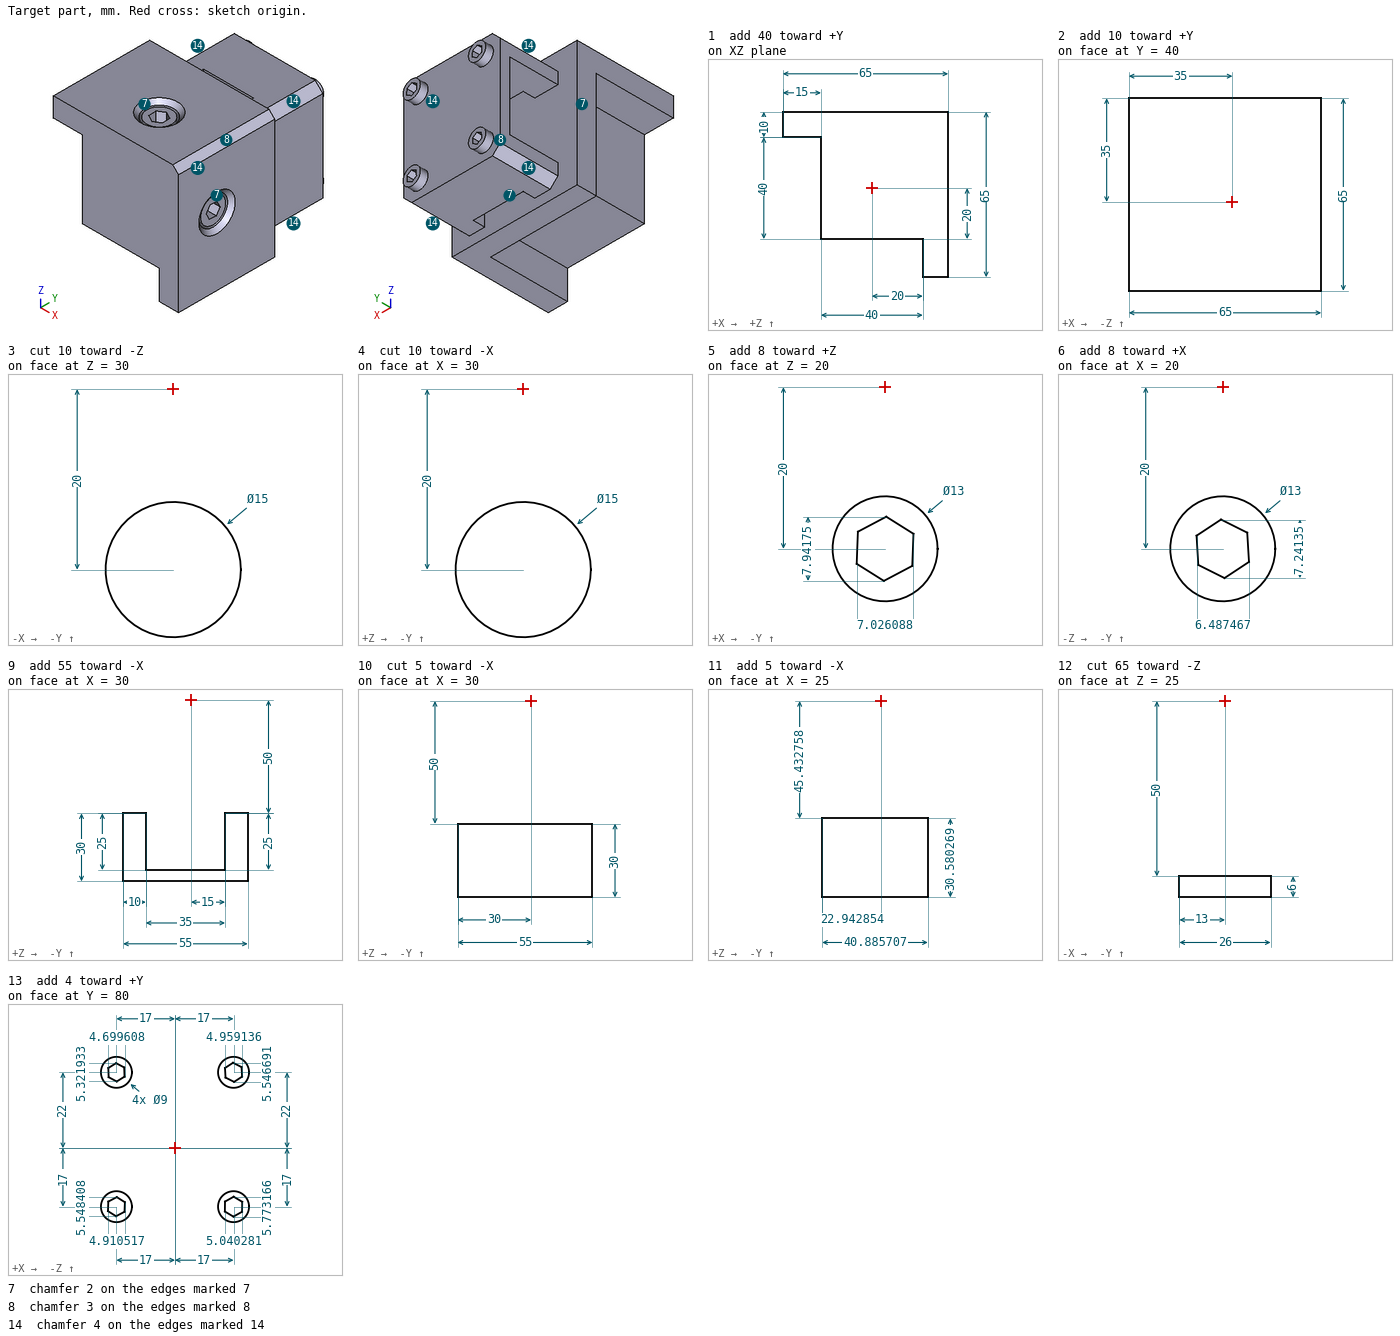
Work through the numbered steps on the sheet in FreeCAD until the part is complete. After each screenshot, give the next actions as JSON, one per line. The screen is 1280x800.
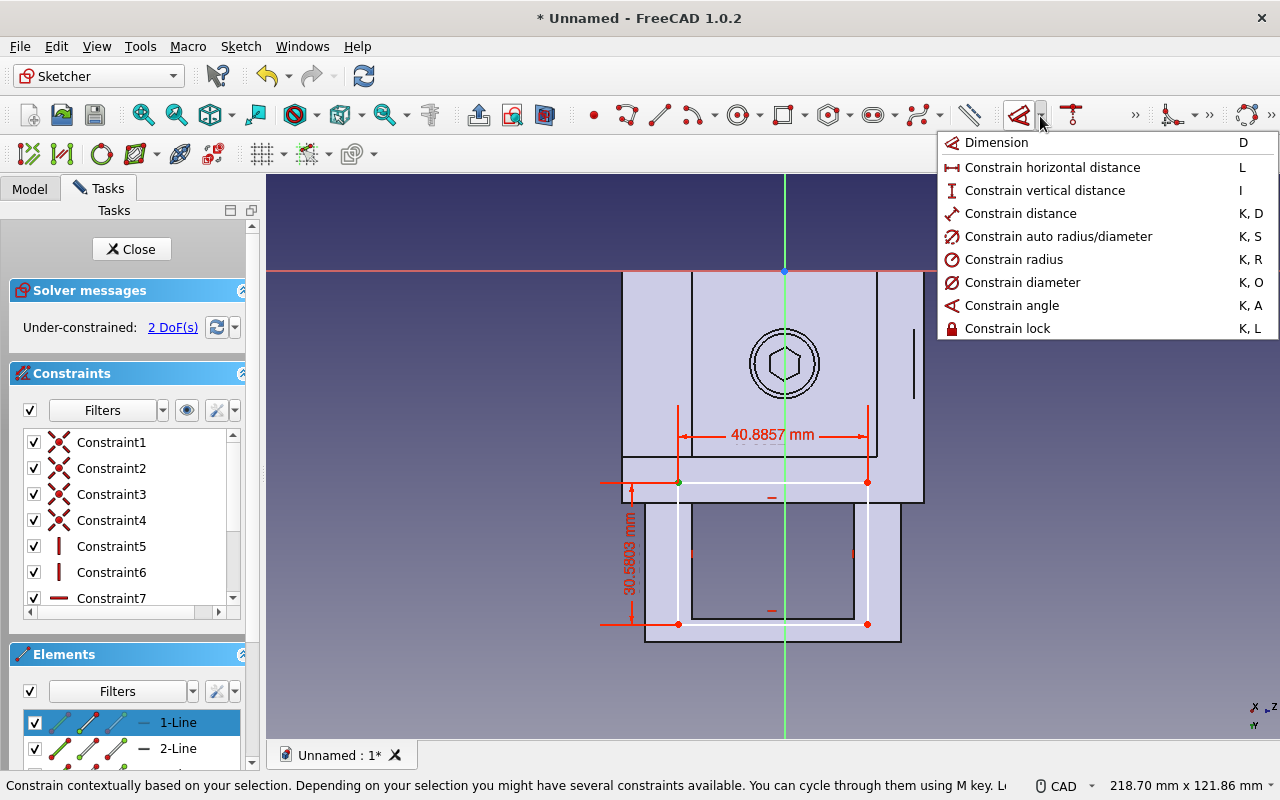
{"action": "left_click", "coordinate": [1108, 168]}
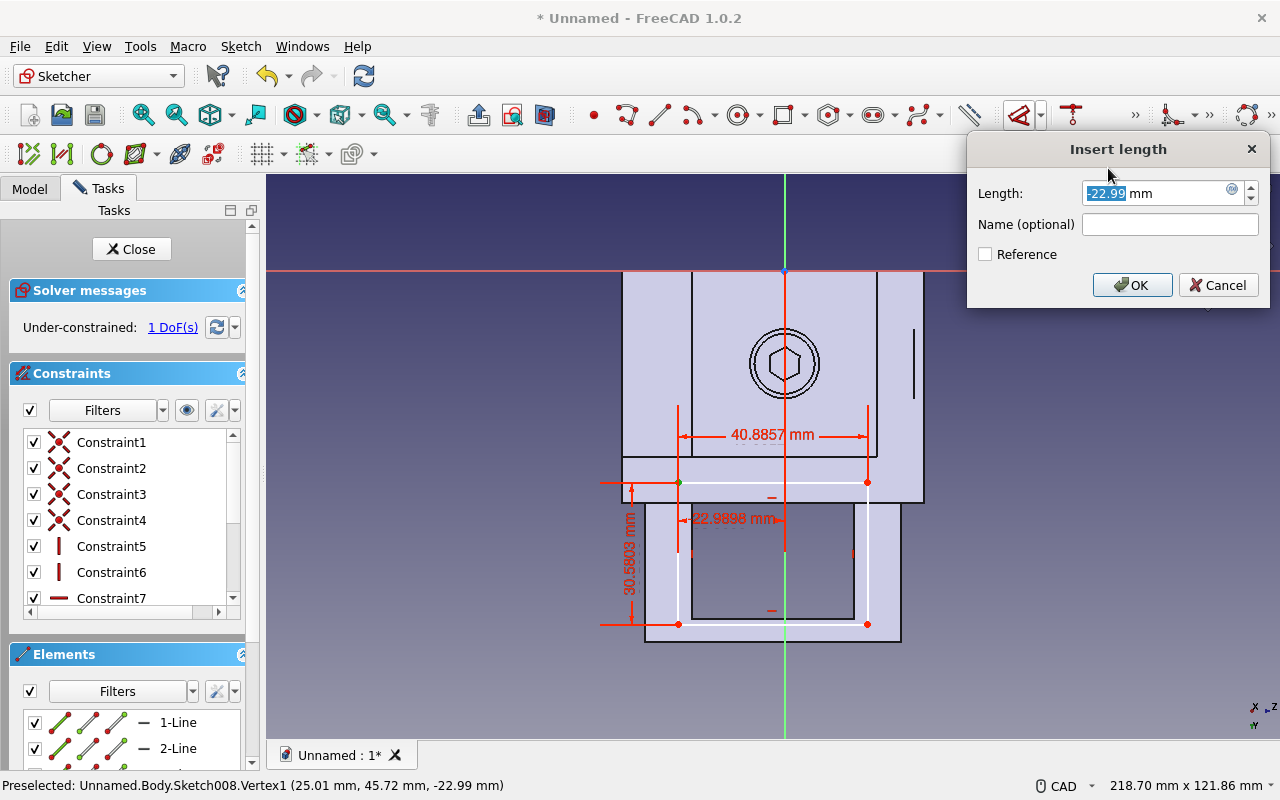
{"action": "type", "text": "-22.942854"}
{"action": "key", "text": "Return"}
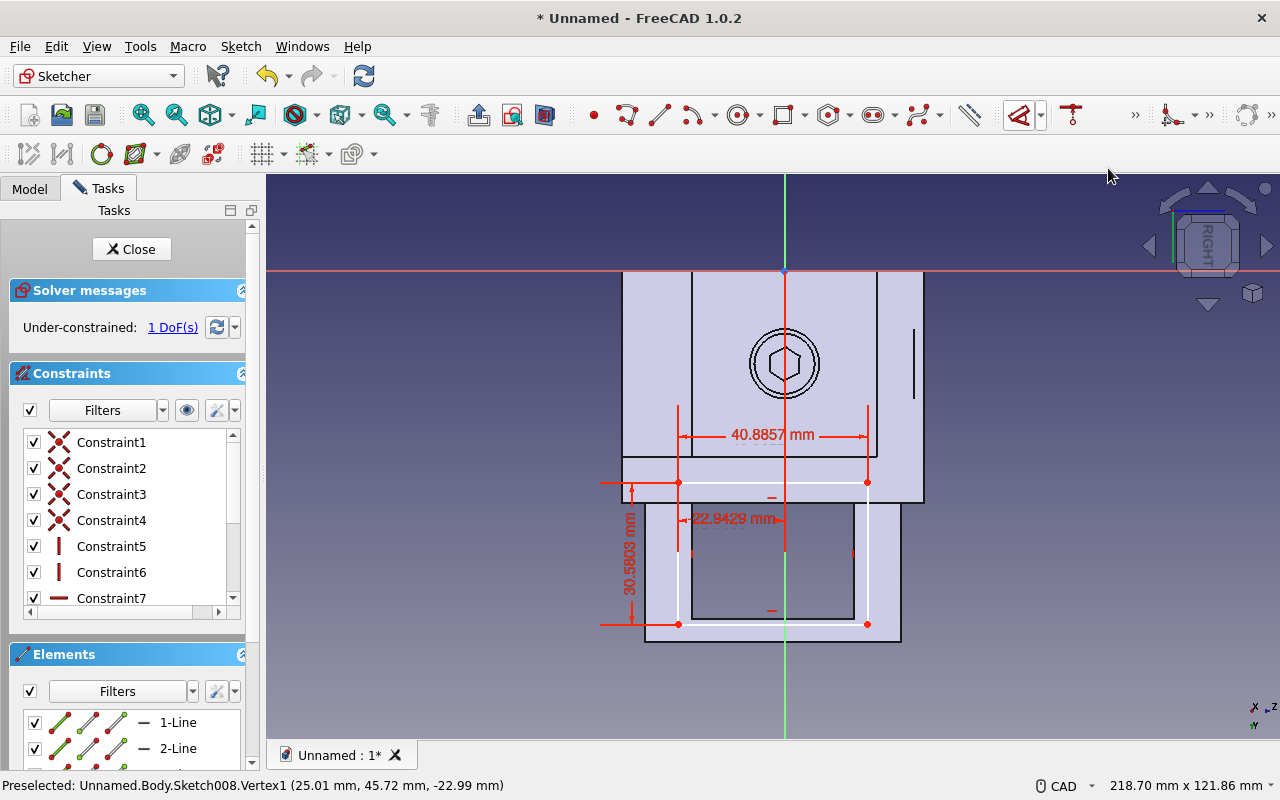
{"action": "left_click", "coordinate": [678, 483]}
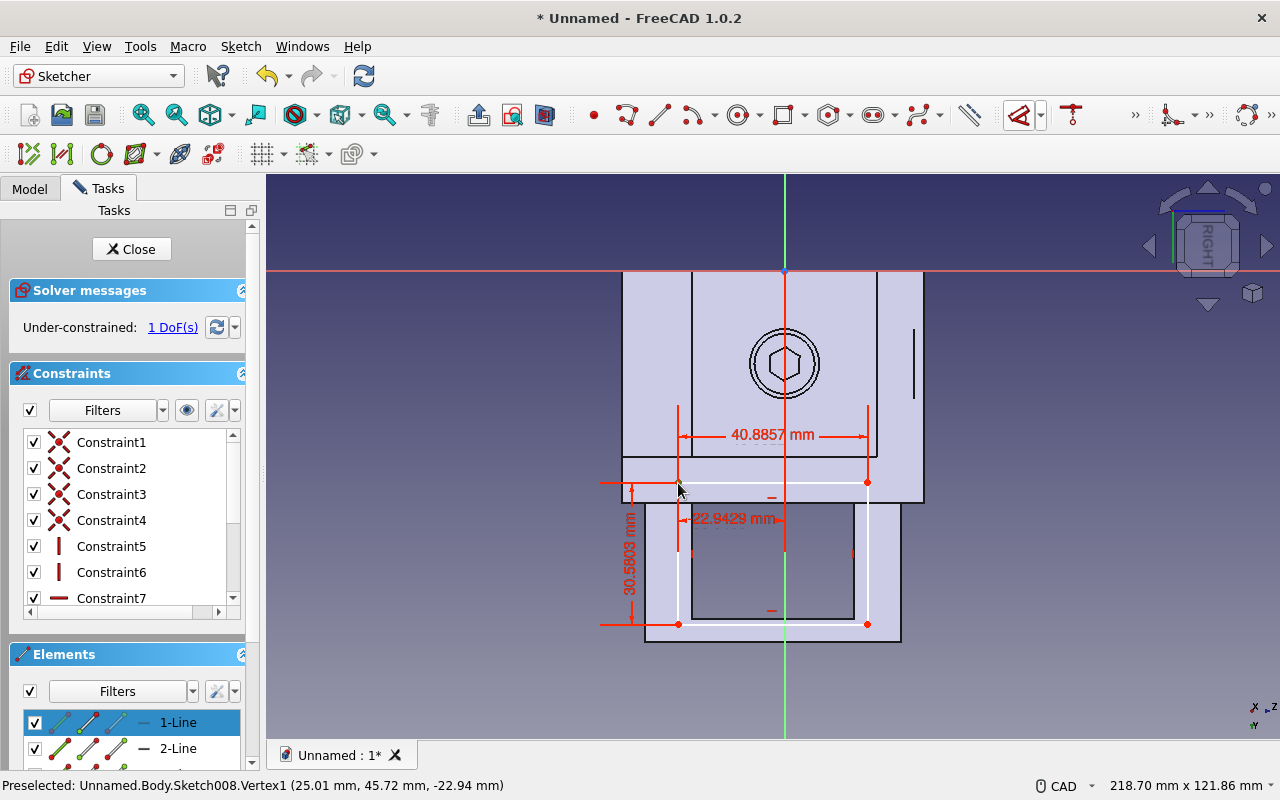
{"action": "left_click", "coordinate": [1040, 116]}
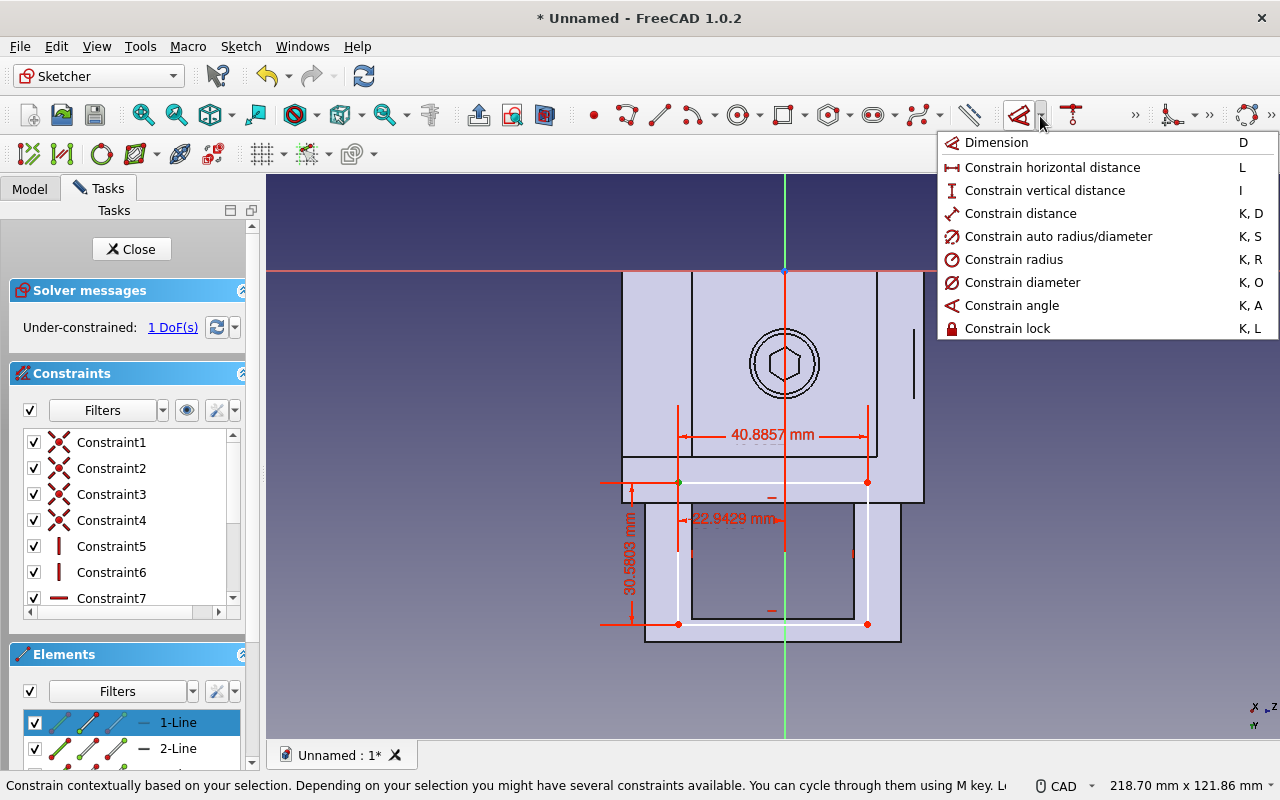
{"action": "left_click", "coordinate": [1108, 190]}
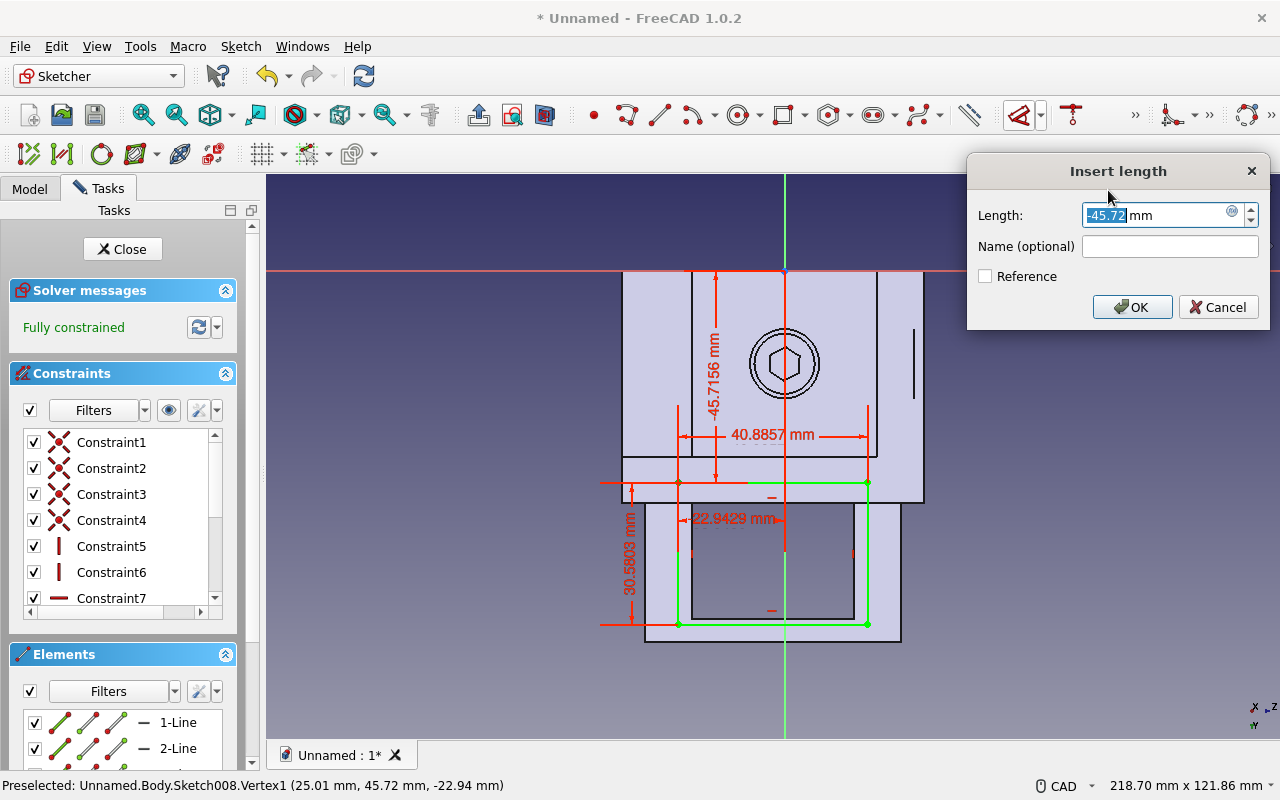
{"action": "type", "text": "-45.432758"}
{"action": "key", "text": "Return"}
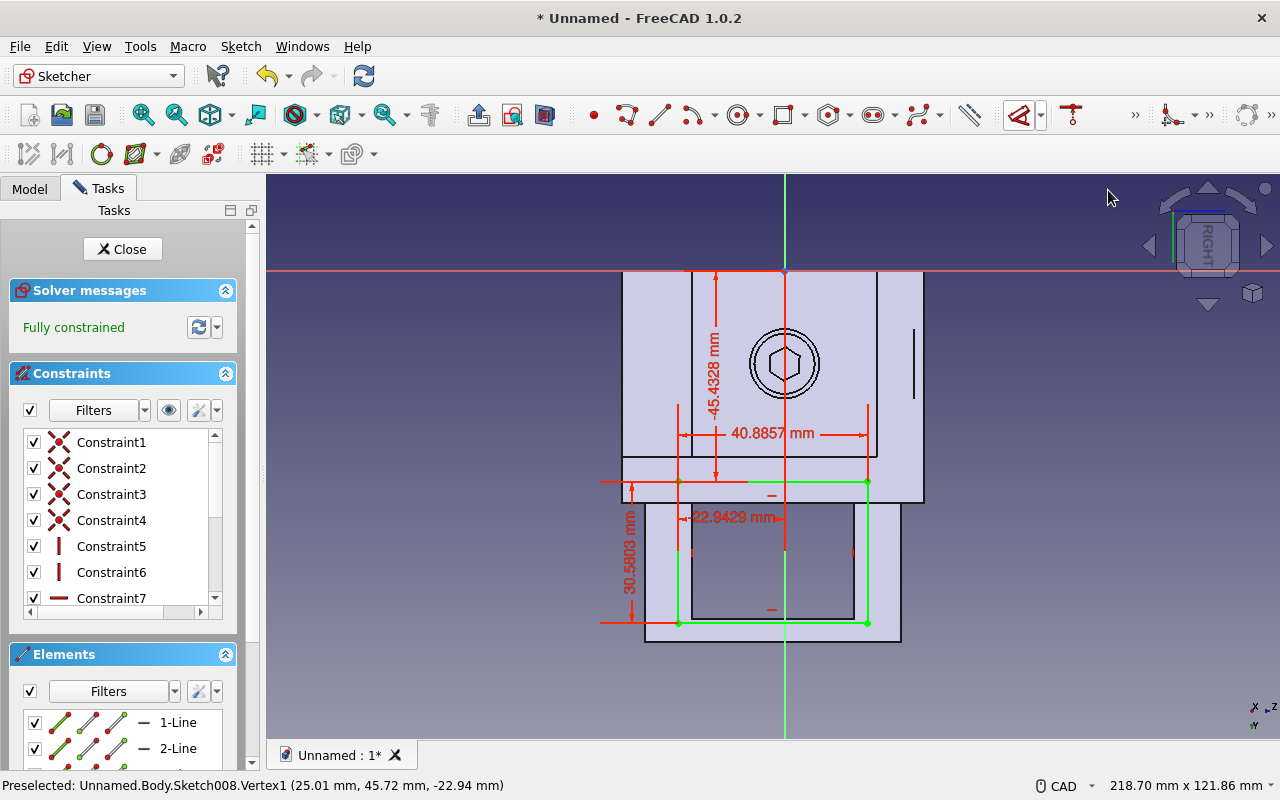
{"action": "left_click", "coordinate": [123, 249]}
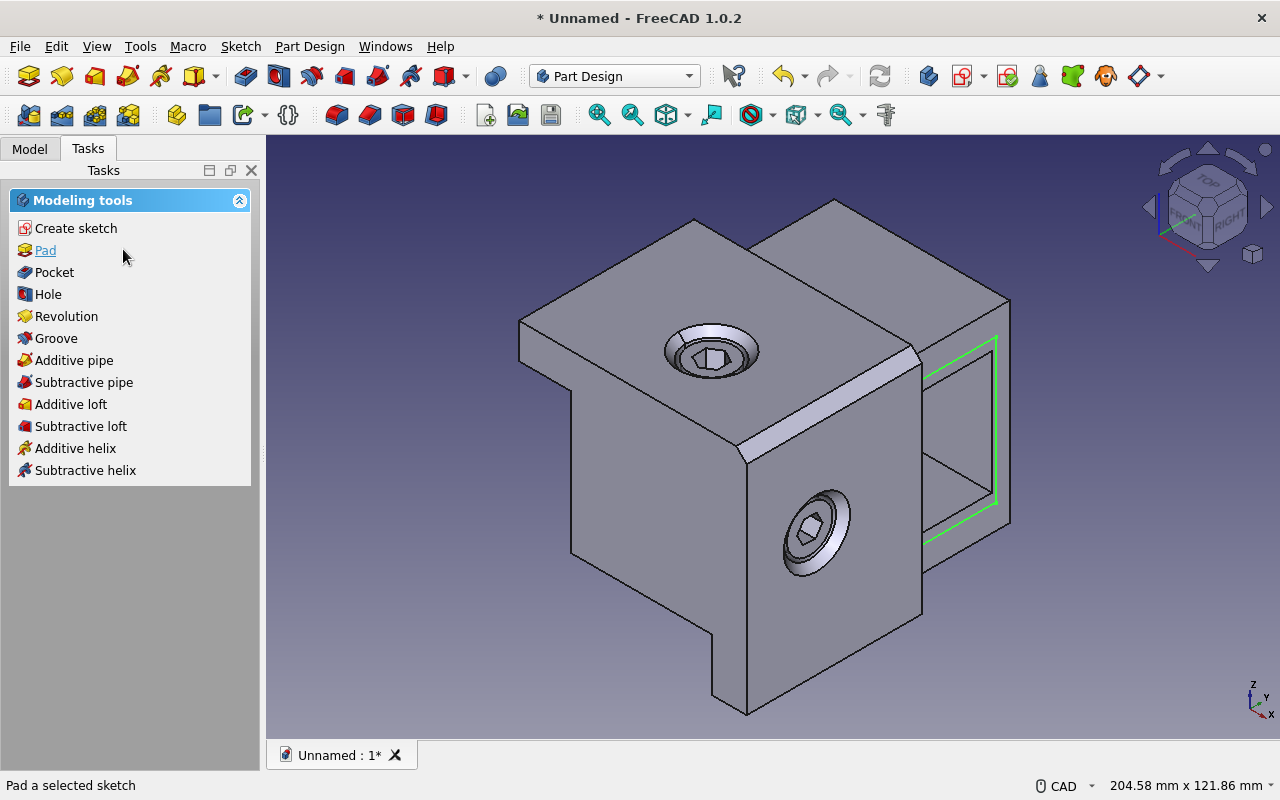
{"action": "left_click", "coordinate": [29, 76]}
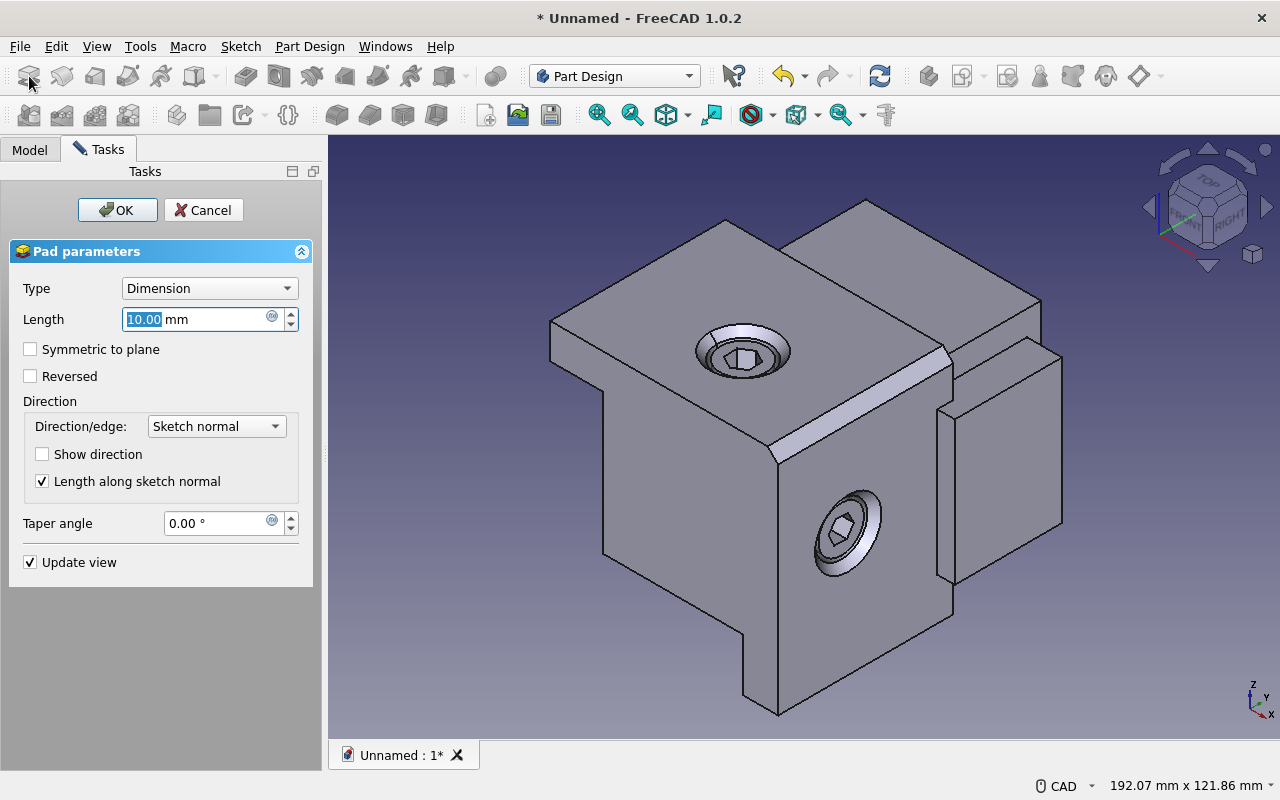
{"action": "type", "text": "5"}
{"action": "key", "text": "Tab"}